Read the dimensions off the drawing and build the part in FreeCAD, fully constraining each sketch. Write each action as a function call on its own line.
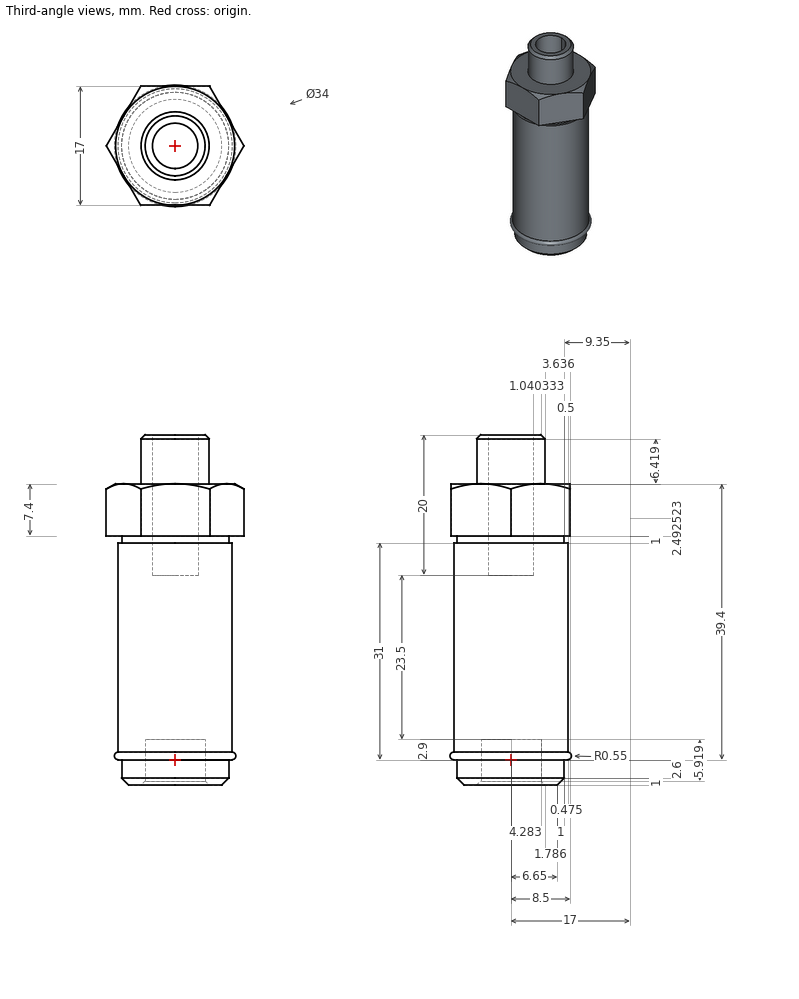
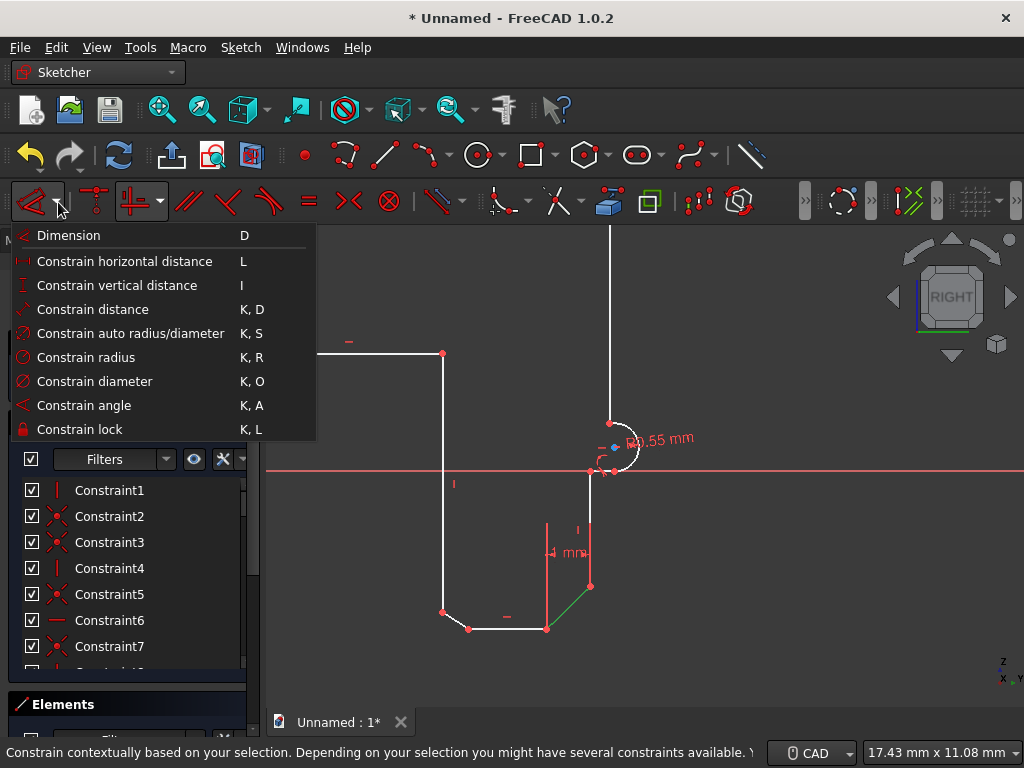
click(164, 285)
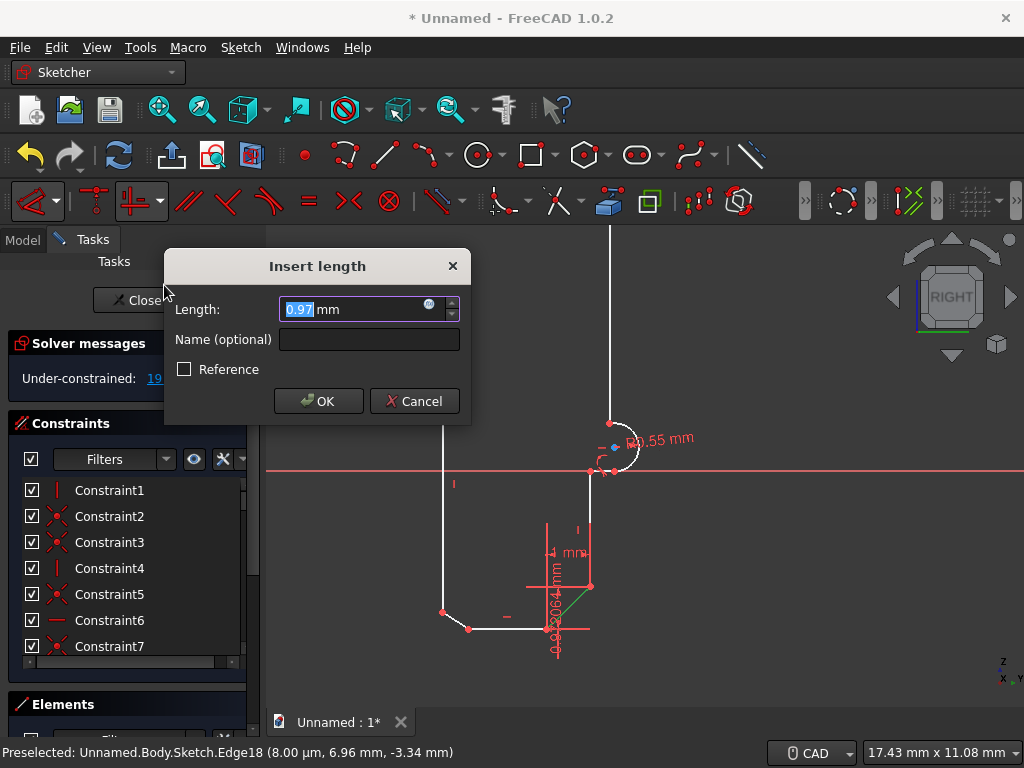
text(1)
key(Return)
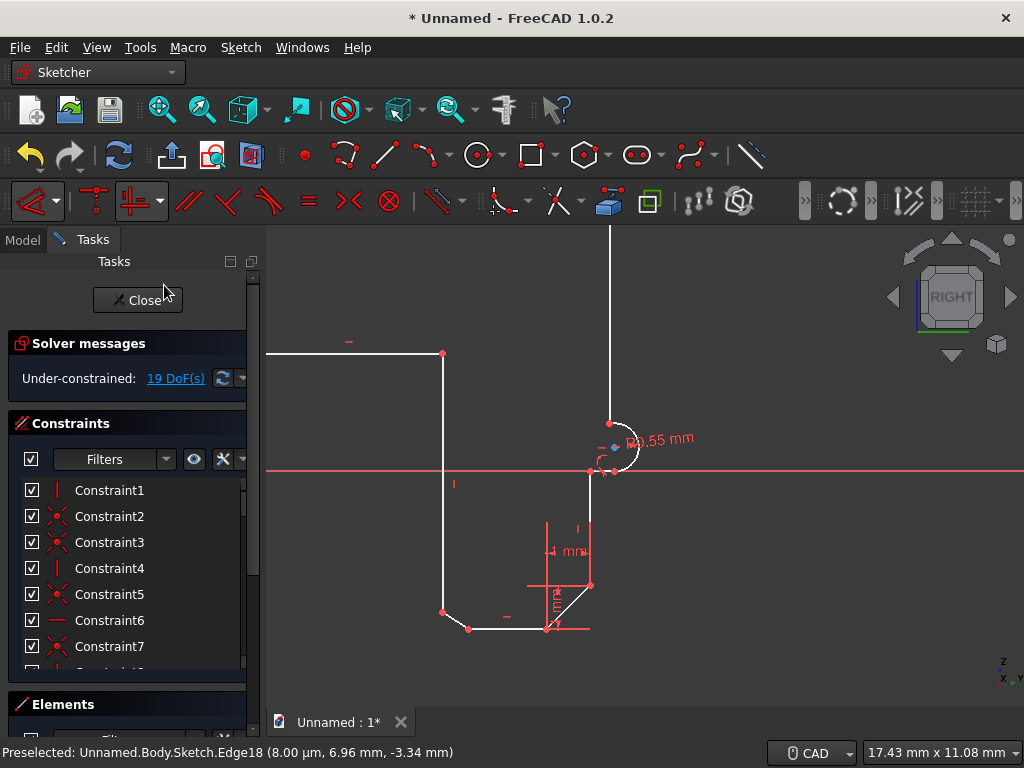
scroll(569, 611, down, 10)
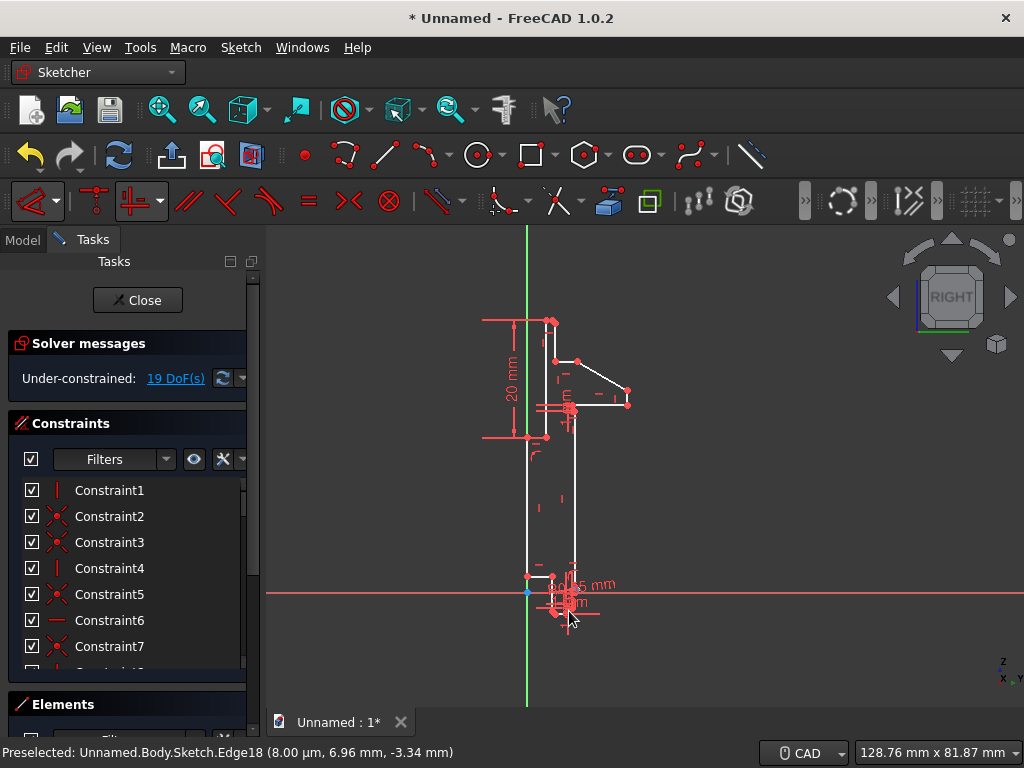
scroll(573, 411, up, 14)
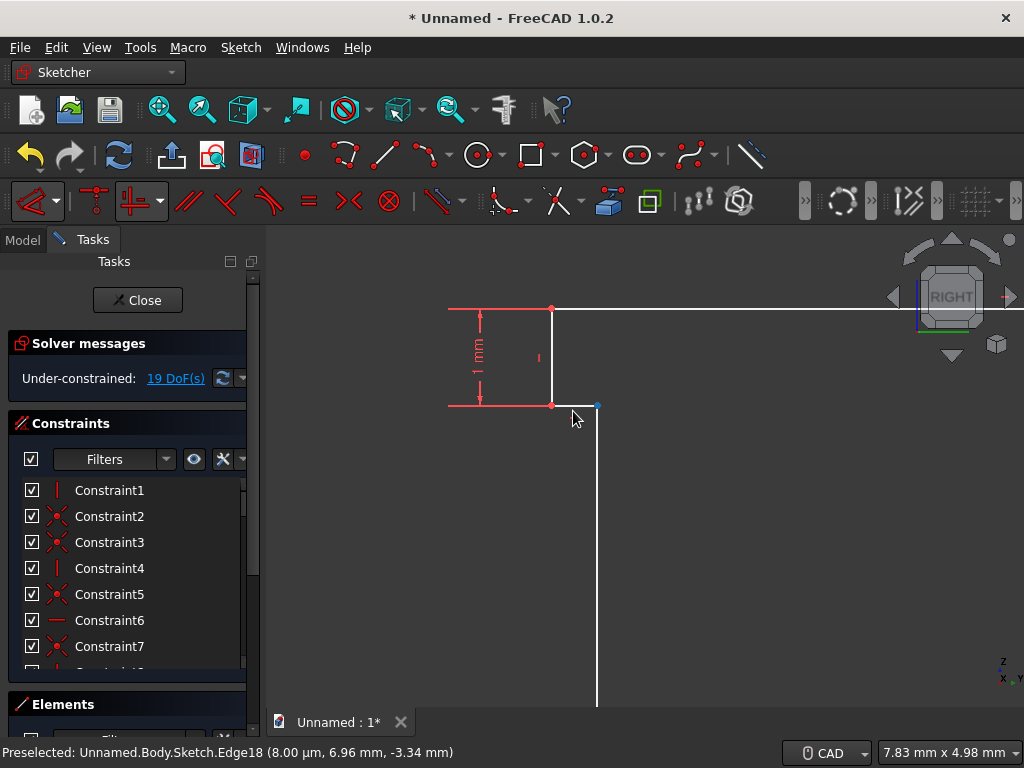
click(574, 406)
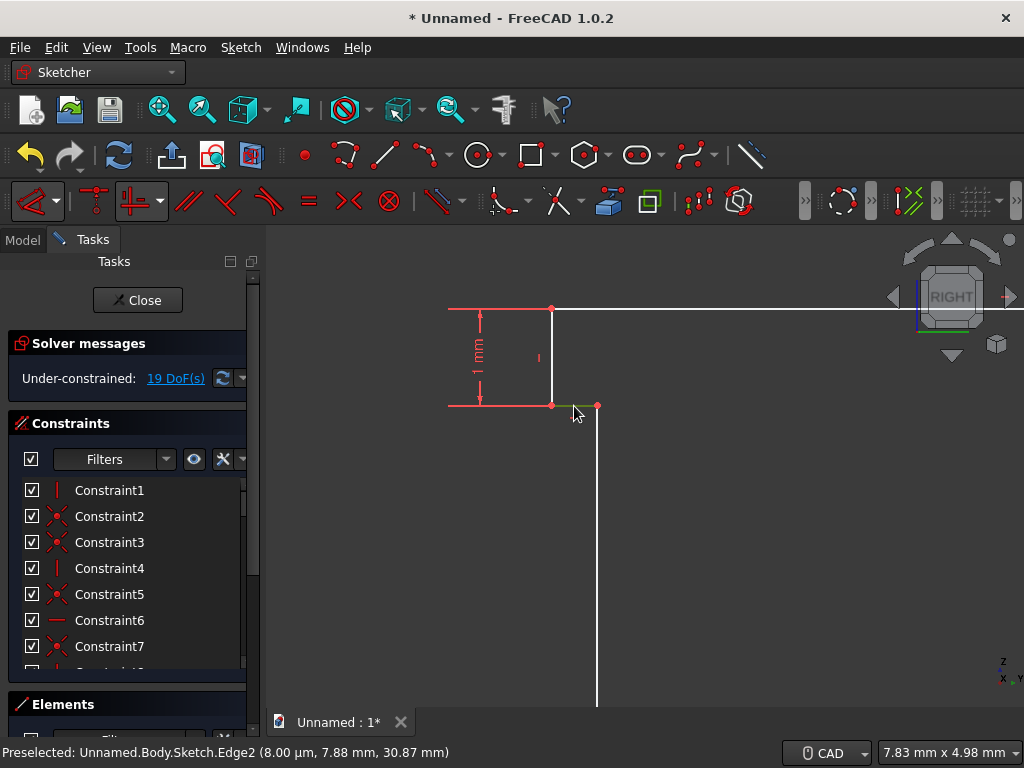
key(l)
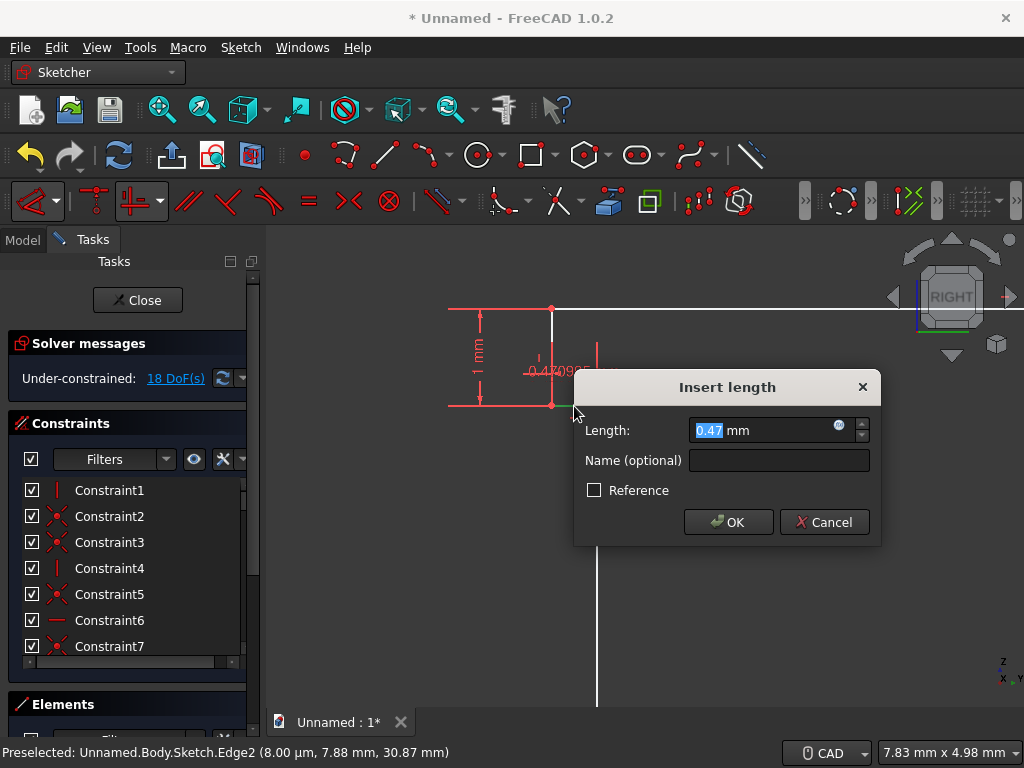
text(0.5)
key(Return)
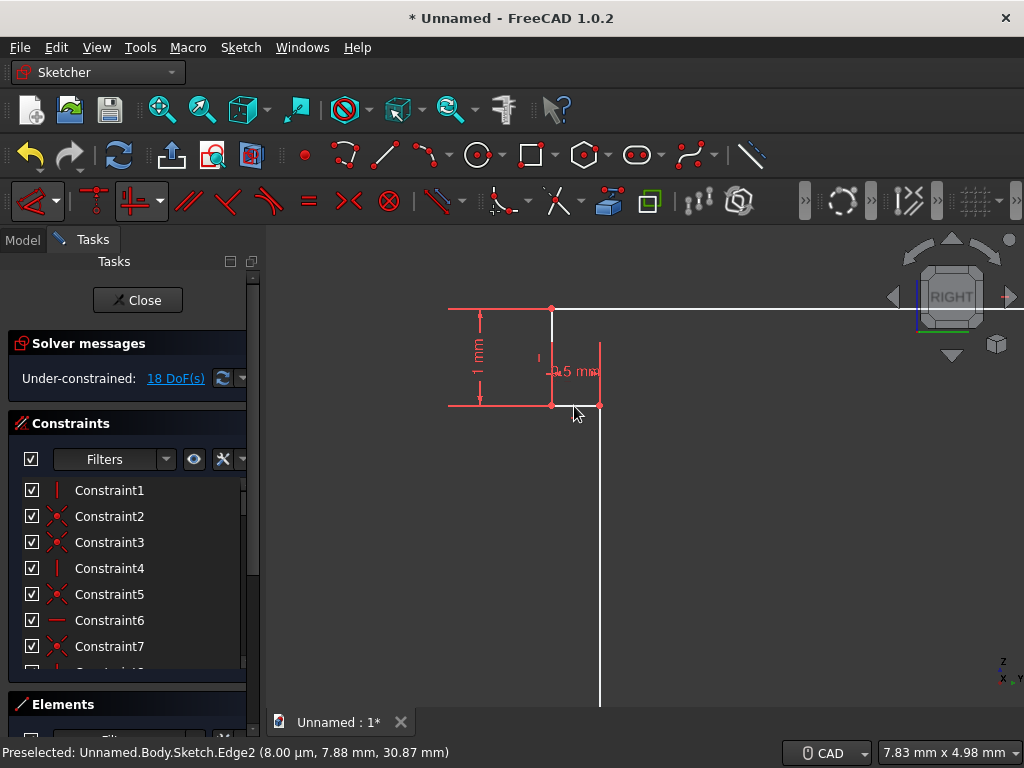
scroll(573, 411, down, 14)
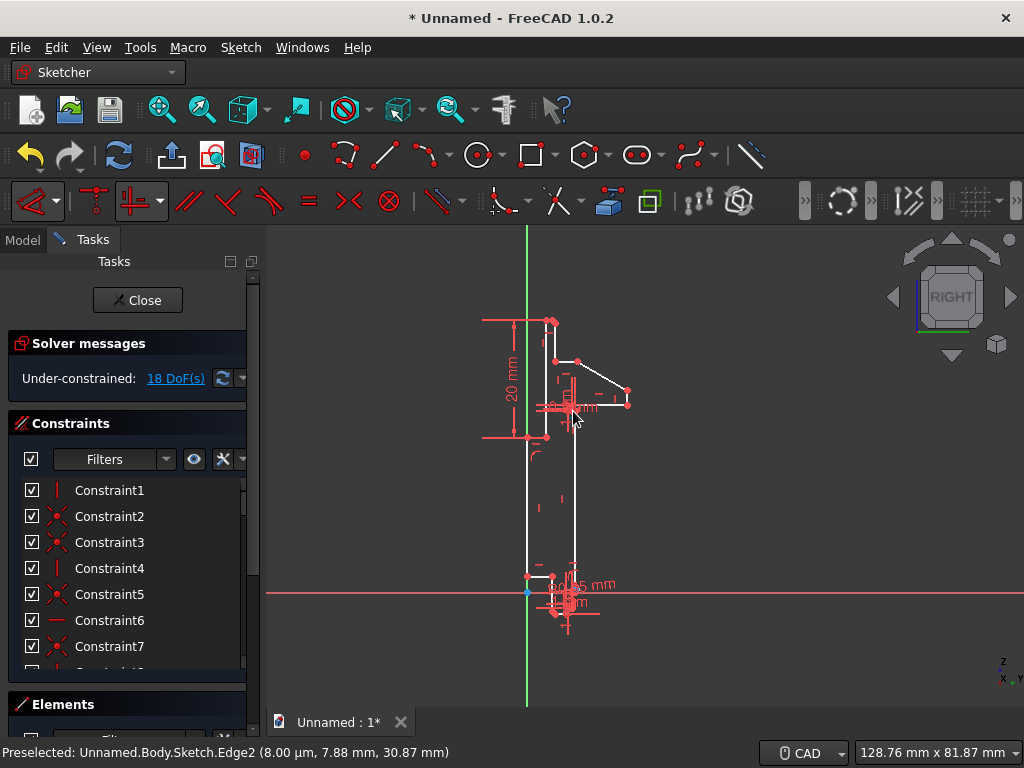
scroll(572, 604, up, 6)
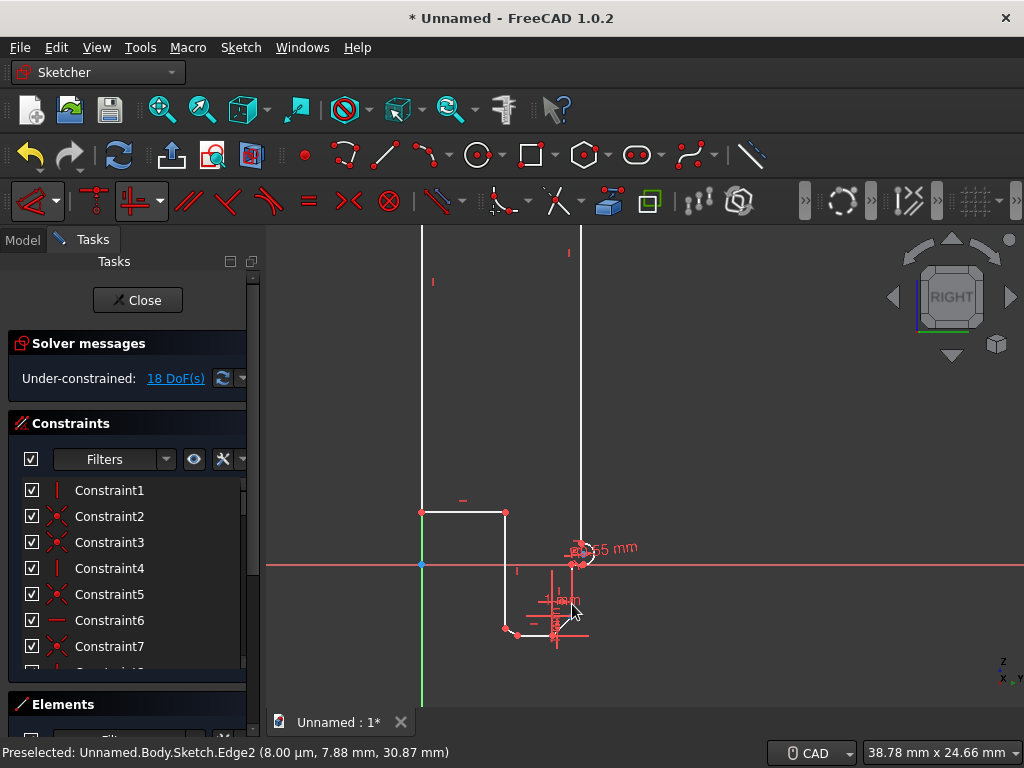
click(572, 580)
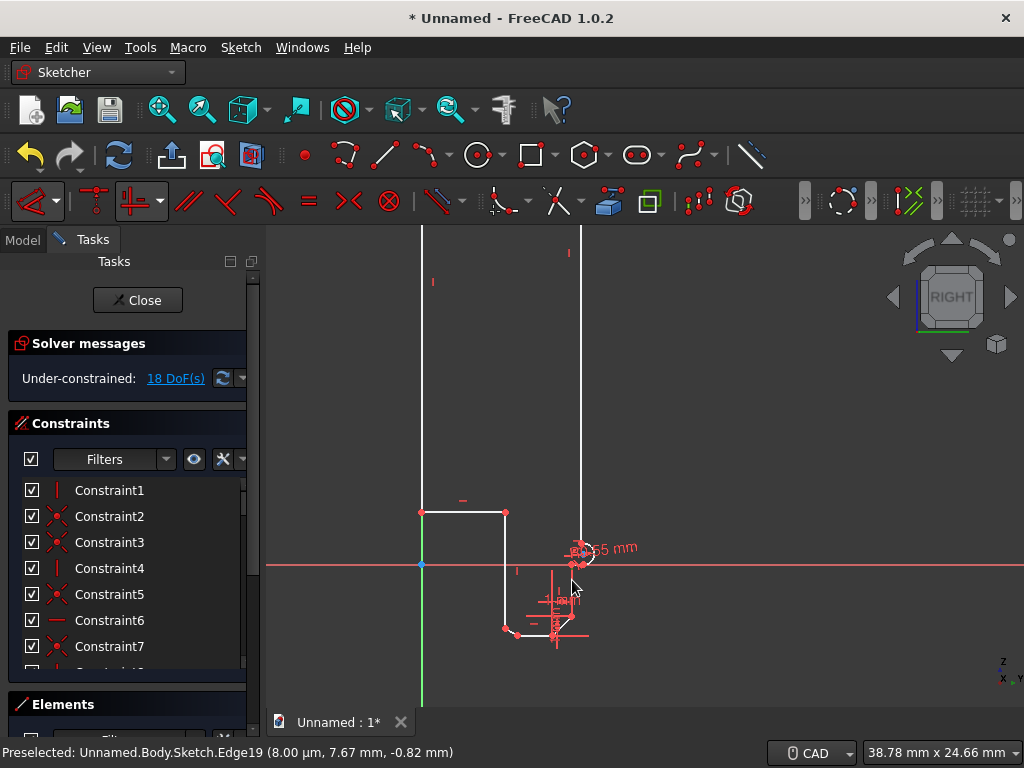
click(58, 202)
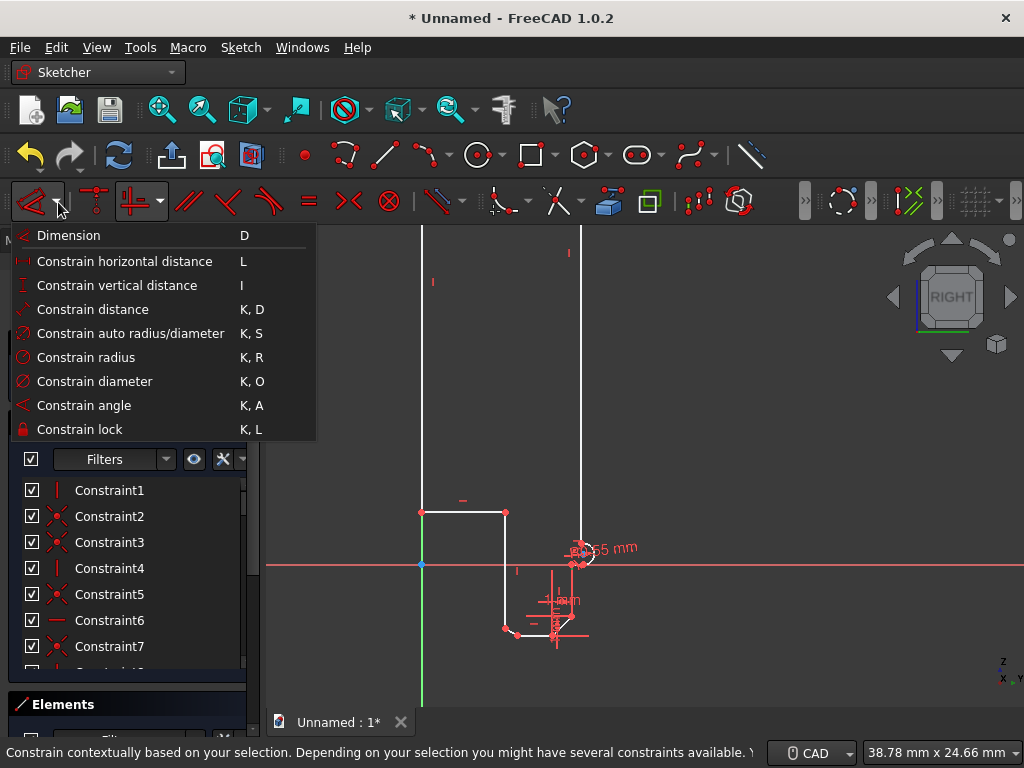
click(164, 285)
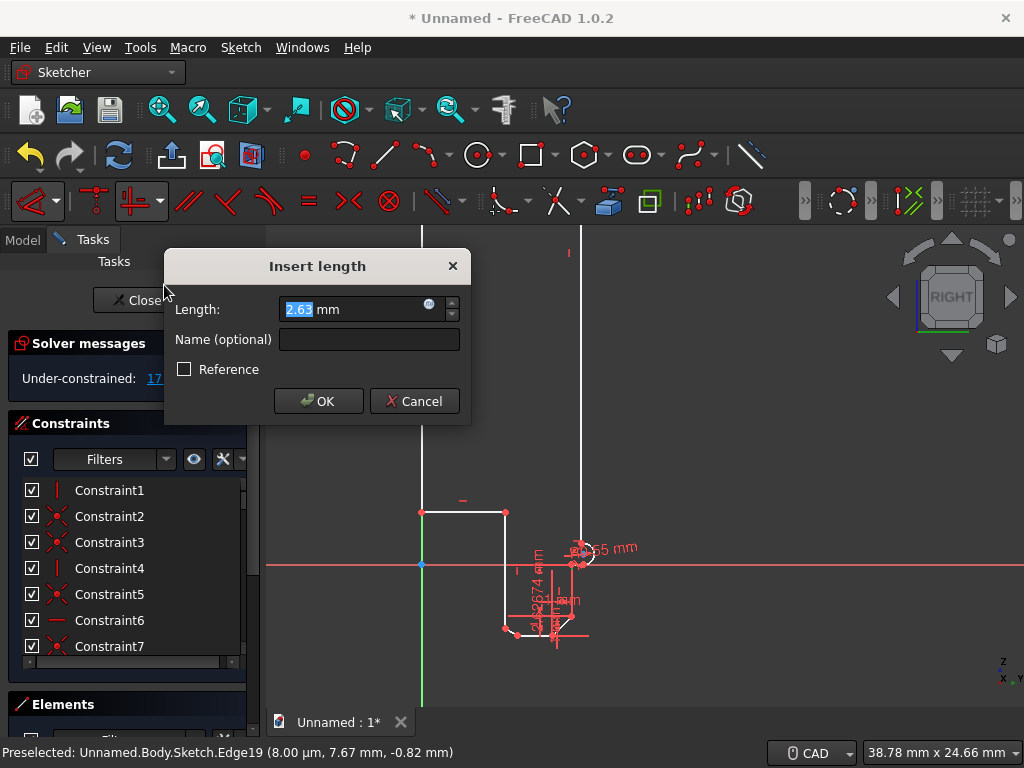
text(2.6)
key(Return)